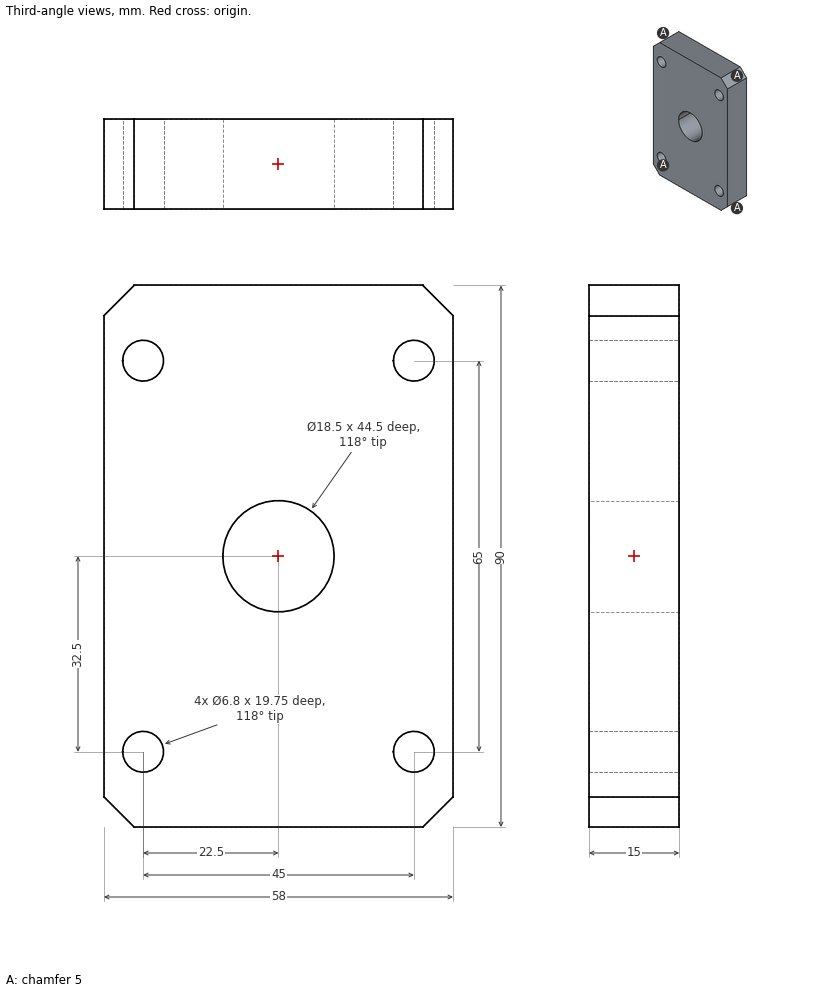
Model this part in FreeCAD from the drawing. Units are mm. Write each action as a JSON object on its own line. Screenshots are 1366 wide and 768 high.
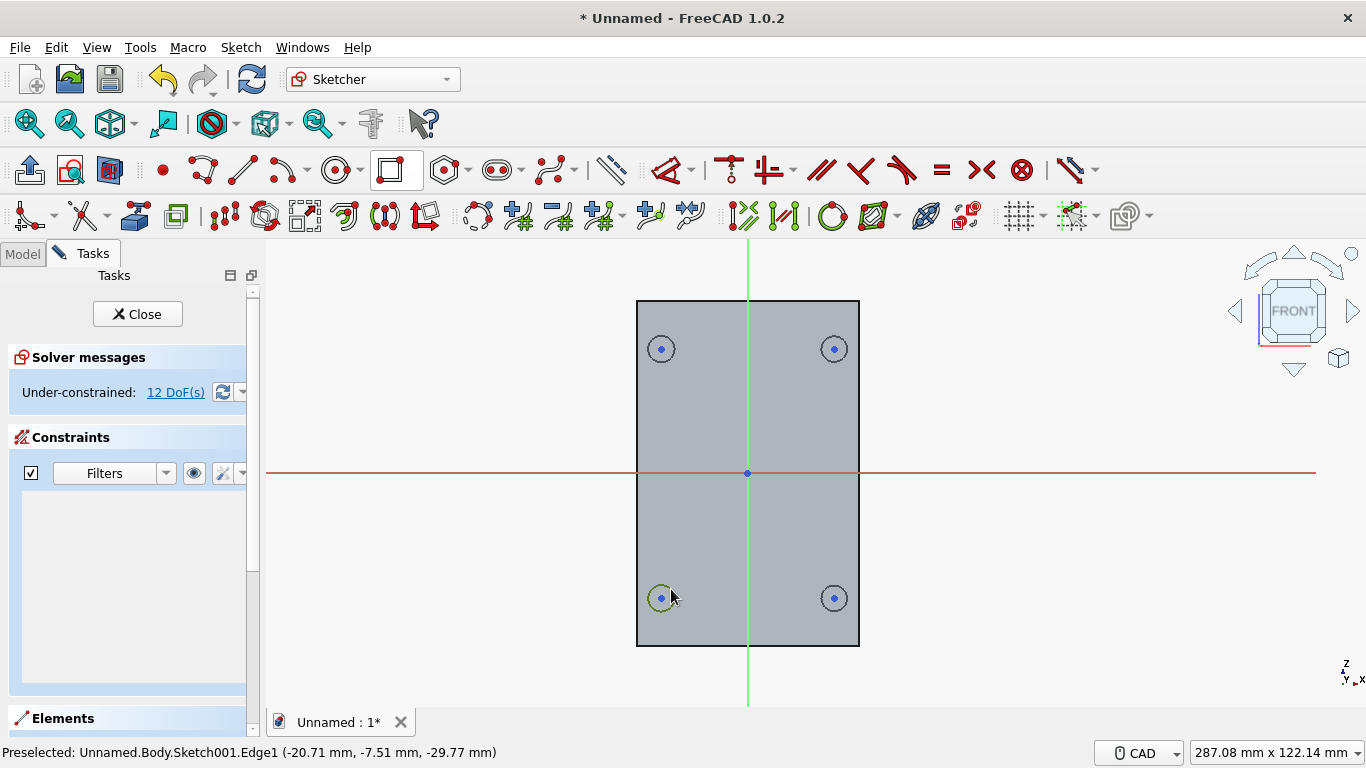
{"action": "left_click", "coordinate": [843, 589]}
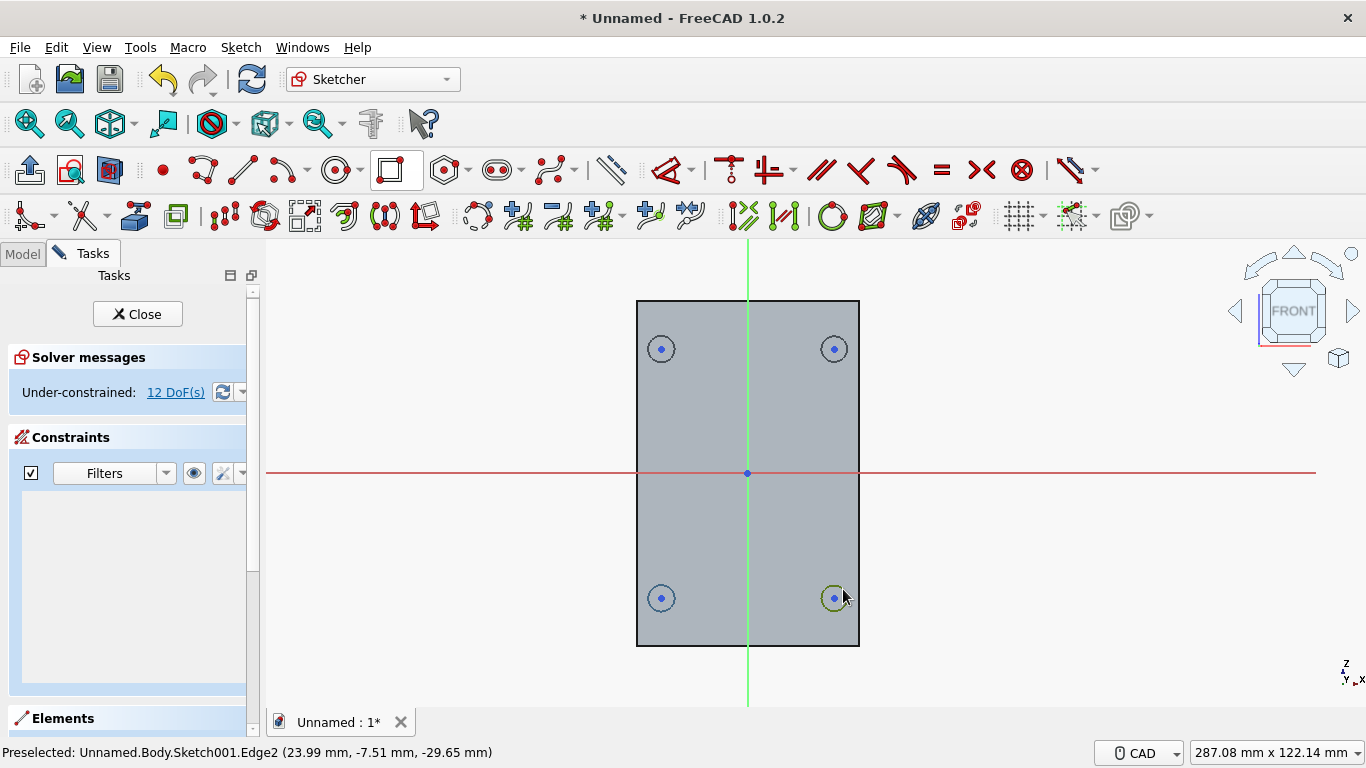
{"action": "left_click", "coordinate": [843, 340]}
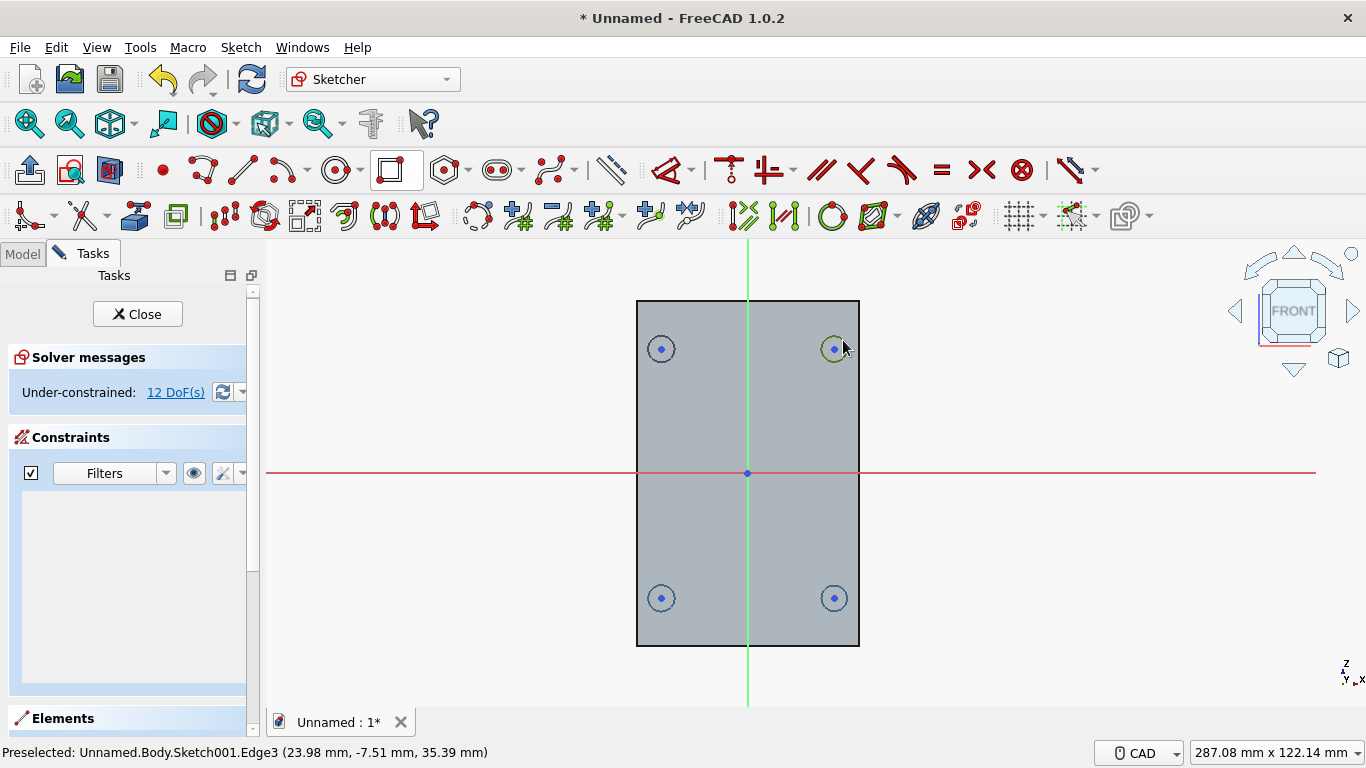
{"action": "left_click", "coordinate": [671, 340]}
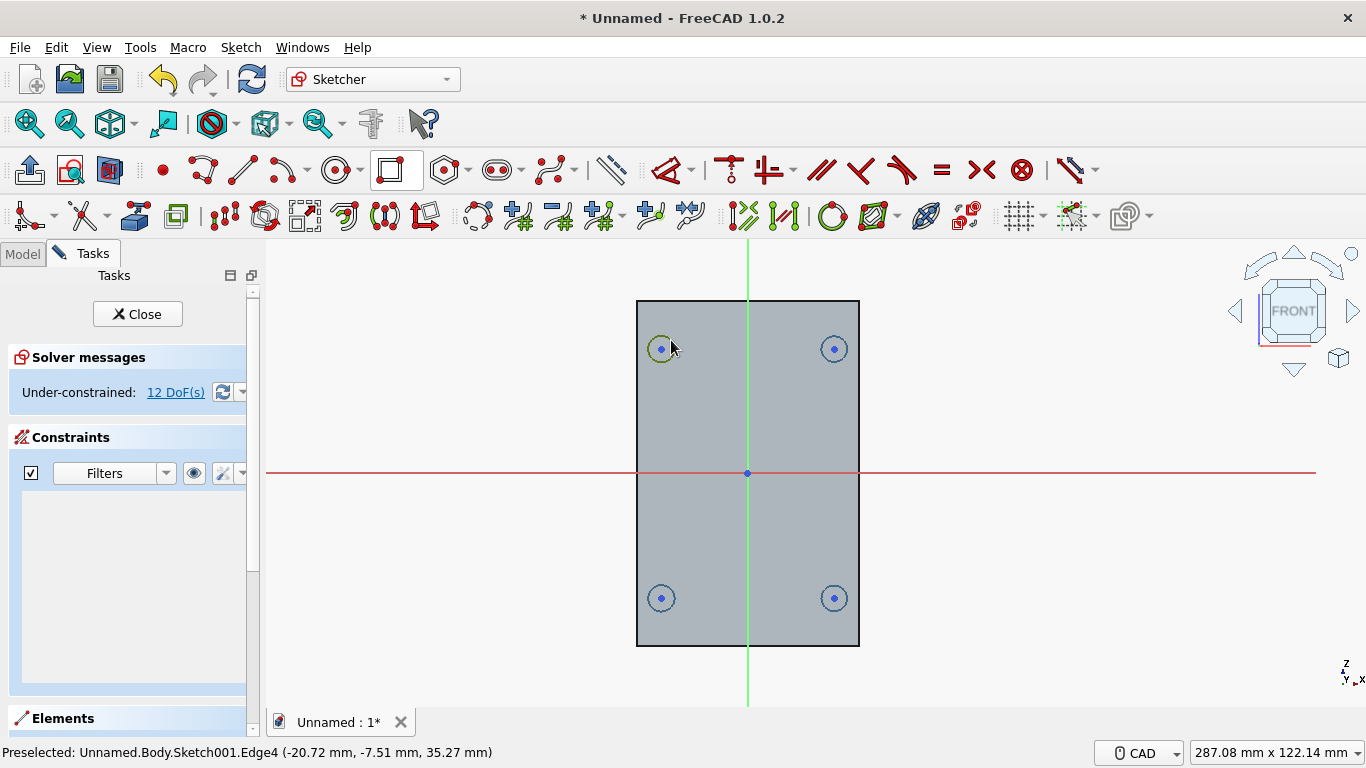
{"action": "left_click", "coordinate": [942, 170]}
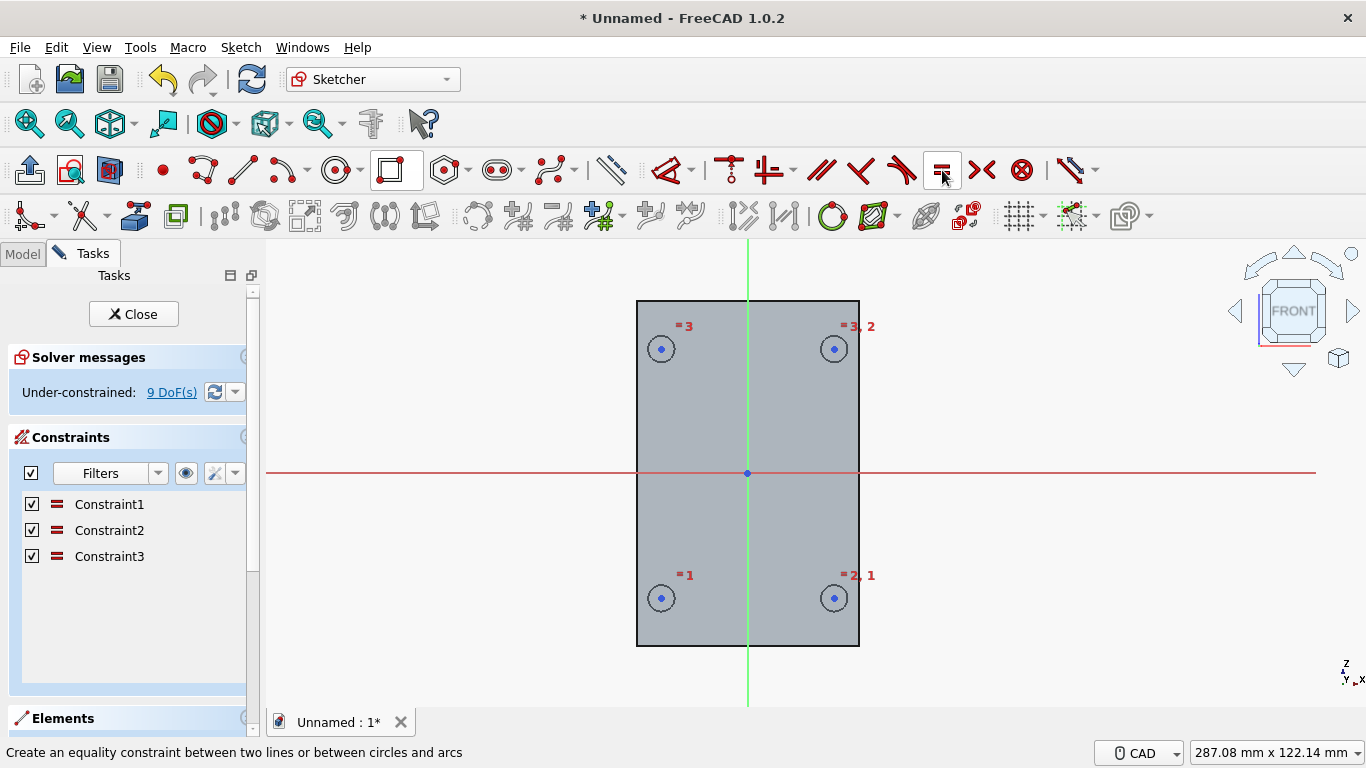
{"action": "key", "text": "d"}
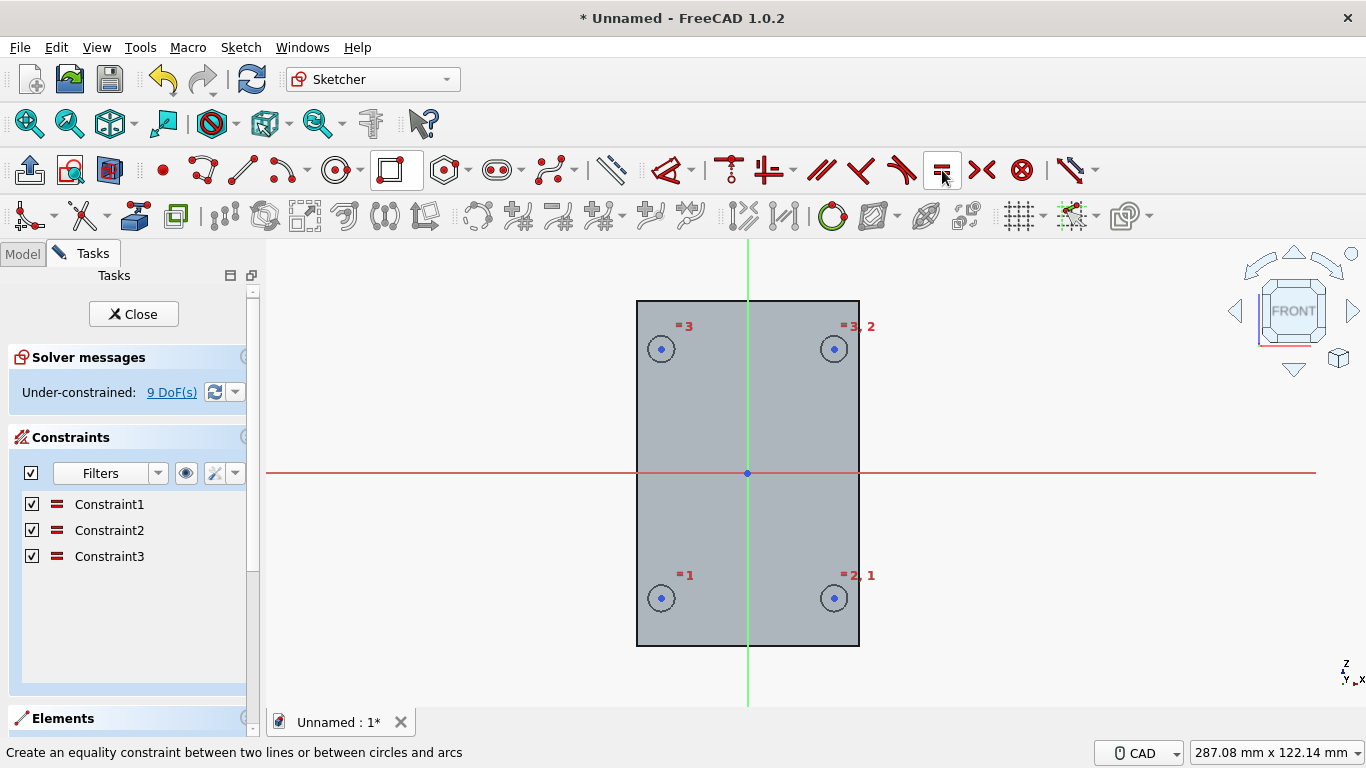
{"action": "scroll", "coordinate": [671, 589], "scroll_direction": "up", "scroll_amount": 3}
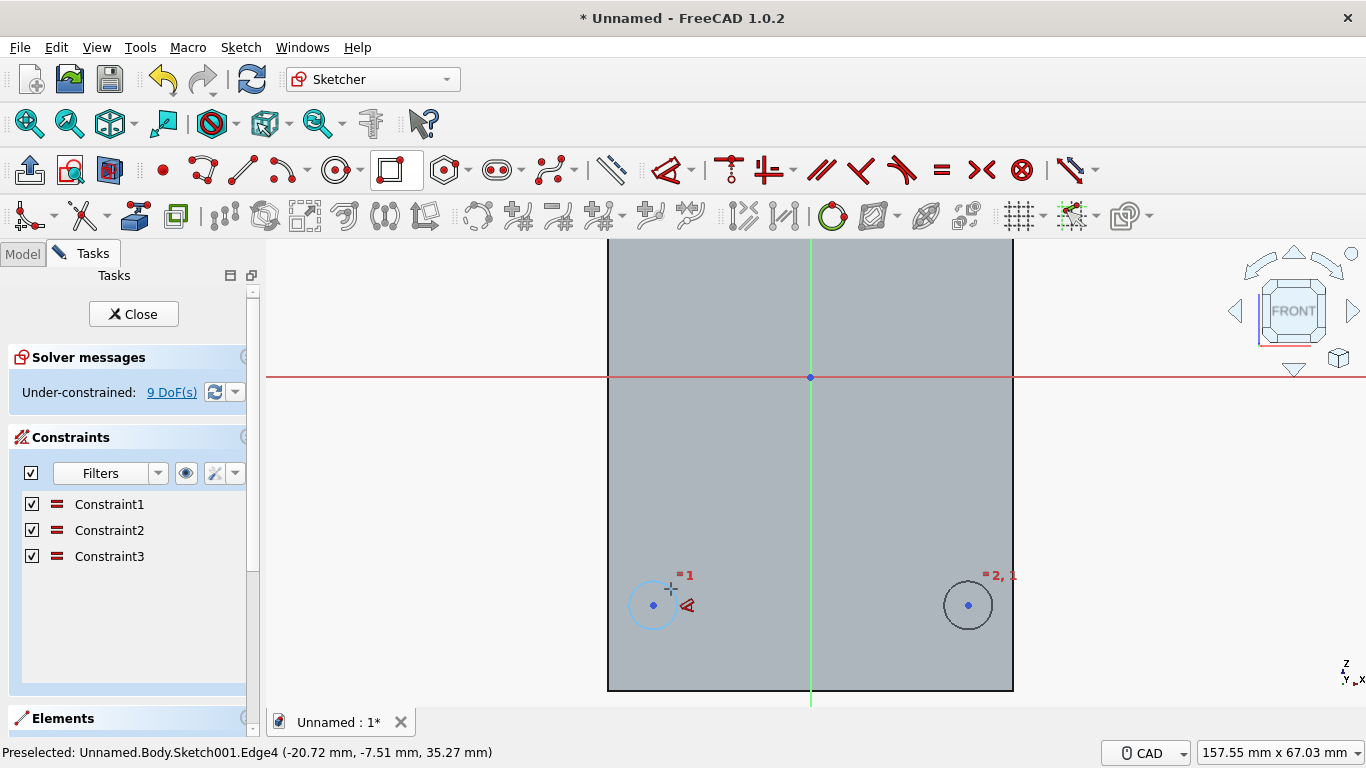
{"action": "left_click", "coordinate": [670, 588]}
{"action": "left_click", "coordinate": [692, 565]}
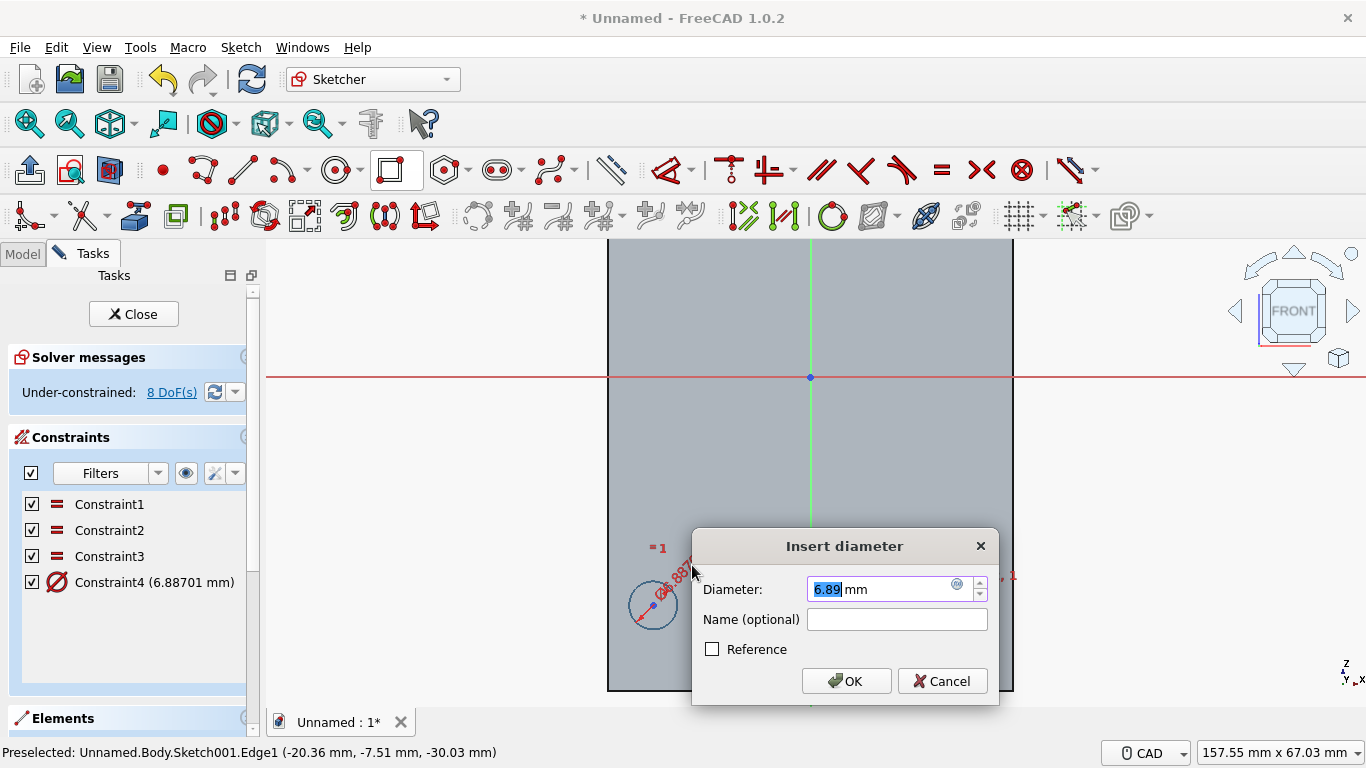
{"action": "type", "text": "6.8"}
{"action": "key", "text": "Return"}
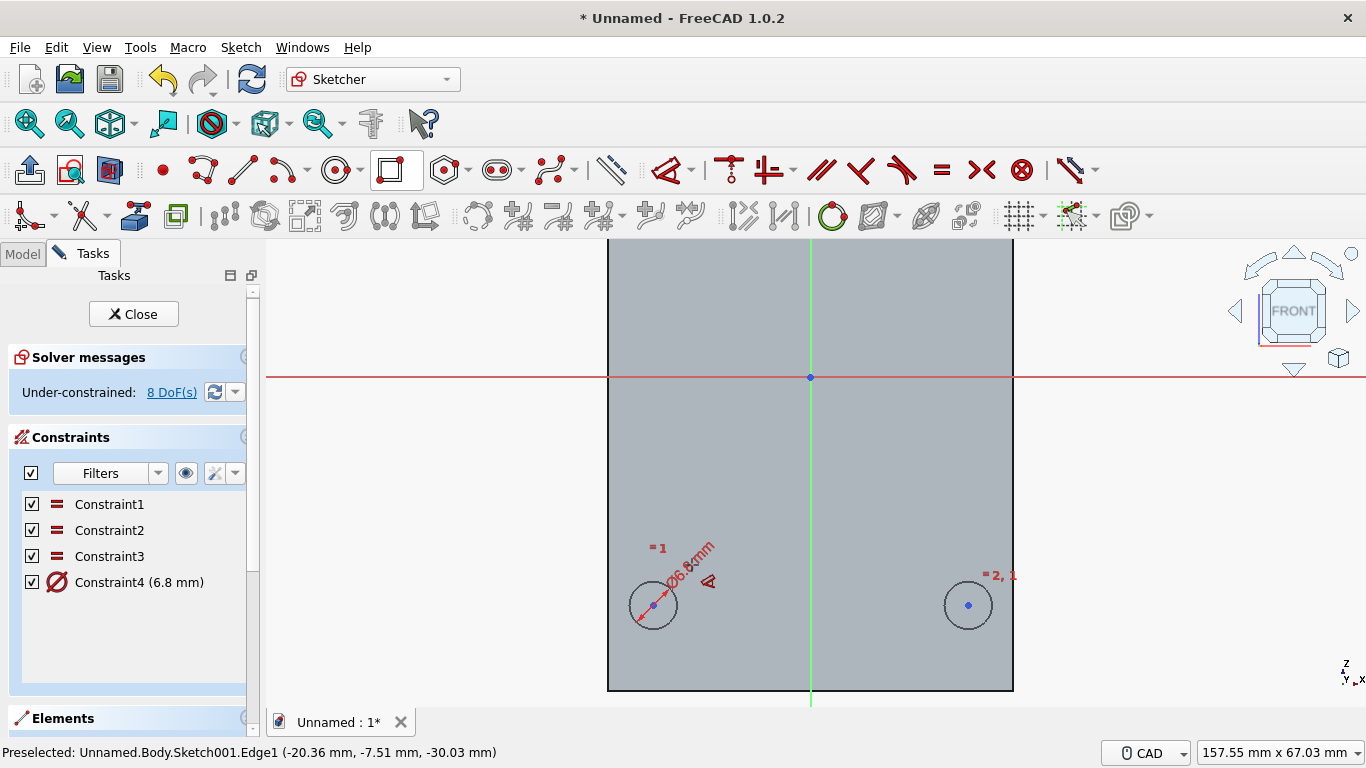
{"action": "left_click", "coordinate": [653, 605]}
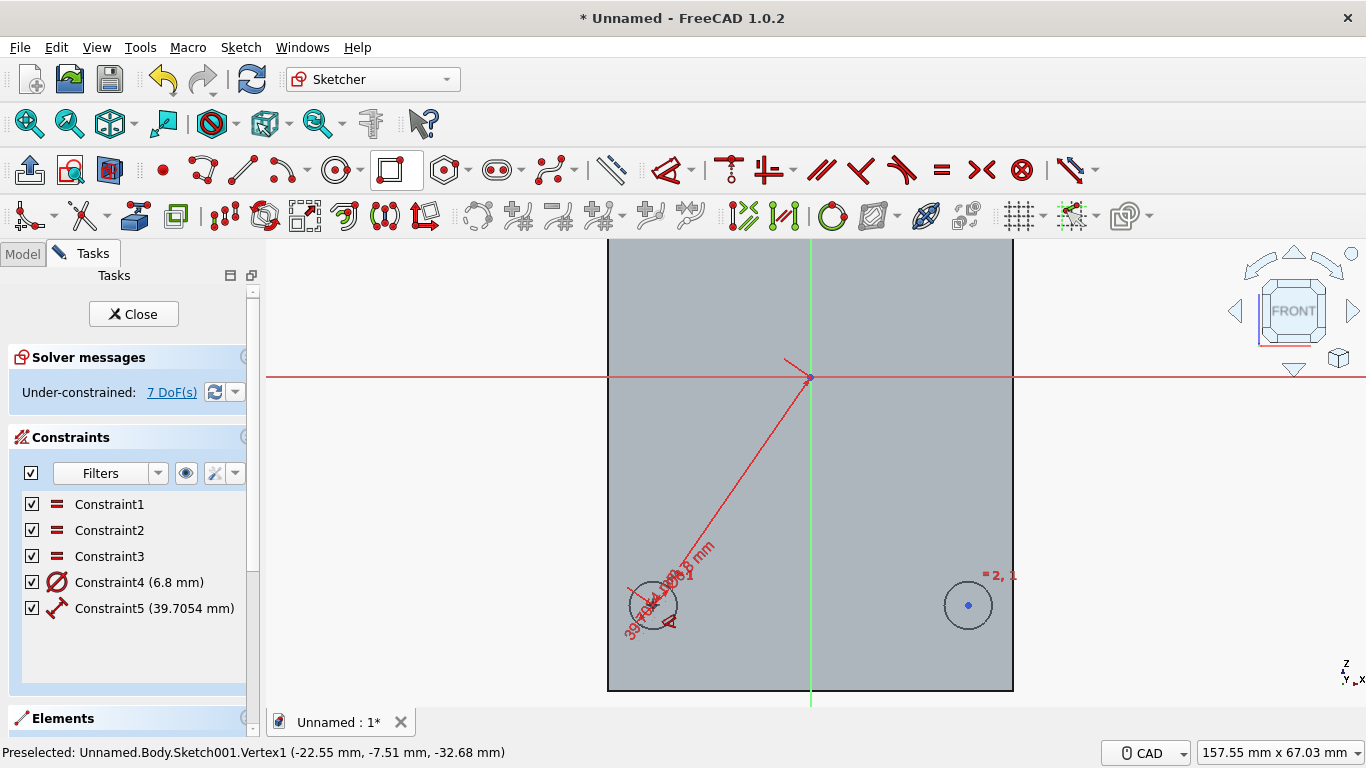
{"action": "left_click", "coordinate": [968, 605]}
{"action": "left_click", "coordinate": [738, 639]}